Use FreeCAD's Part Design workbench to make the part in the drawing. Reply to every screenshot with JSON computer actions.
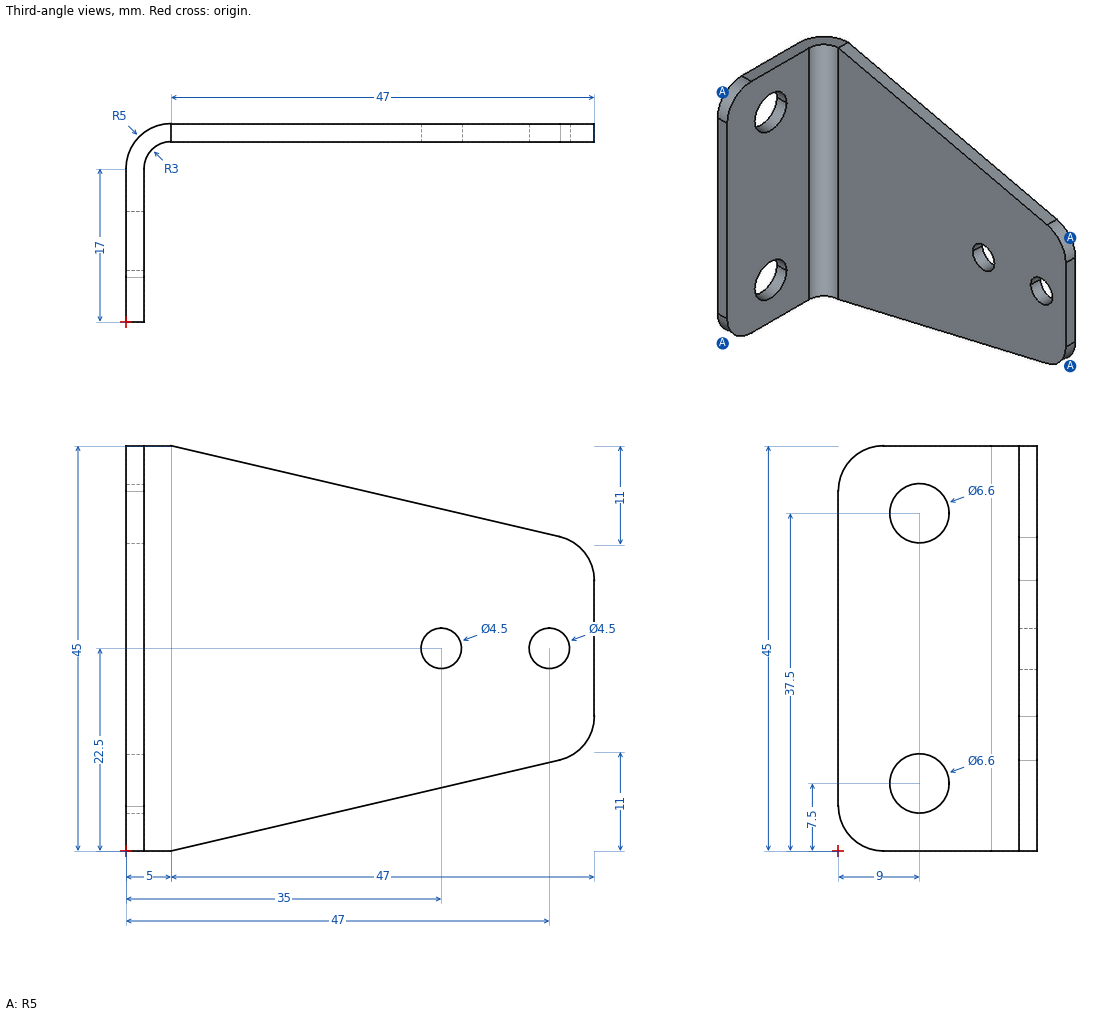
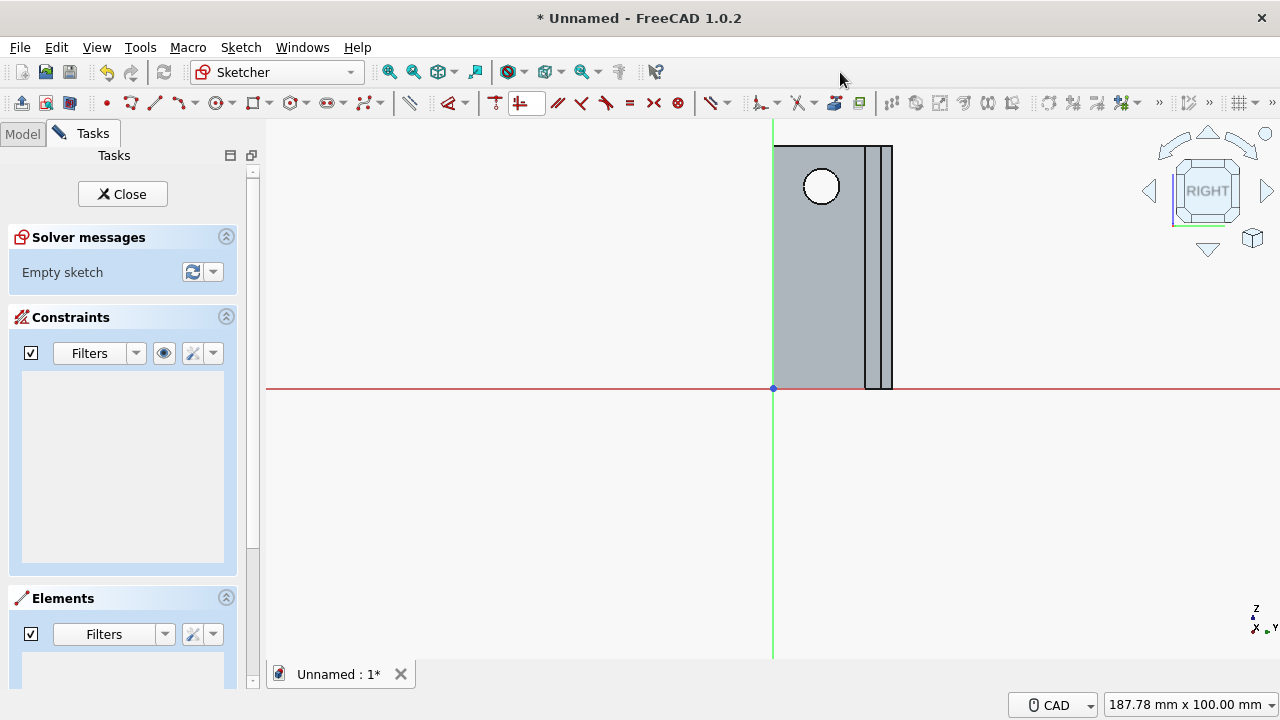
{"action": "scroll", "coordinate": [826, 354], "scroll_direction": "up", "scroll_amount": 9}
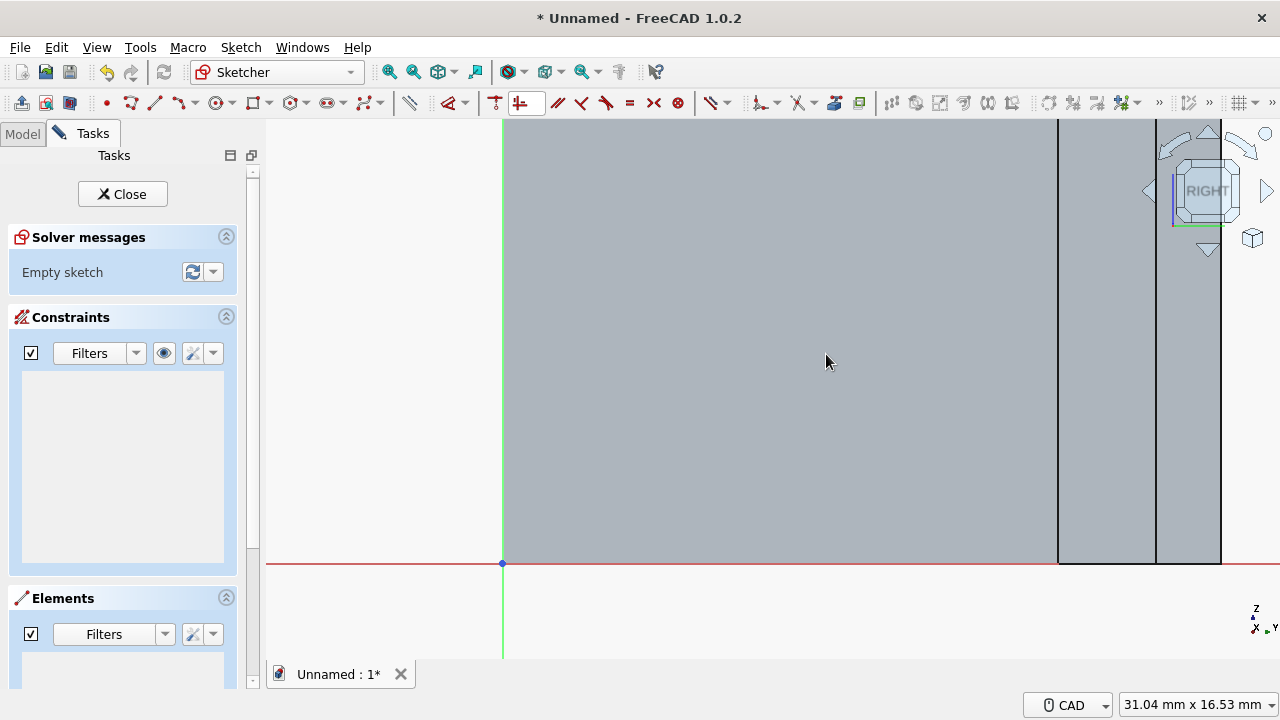
{"action": "key", "text": "g c"}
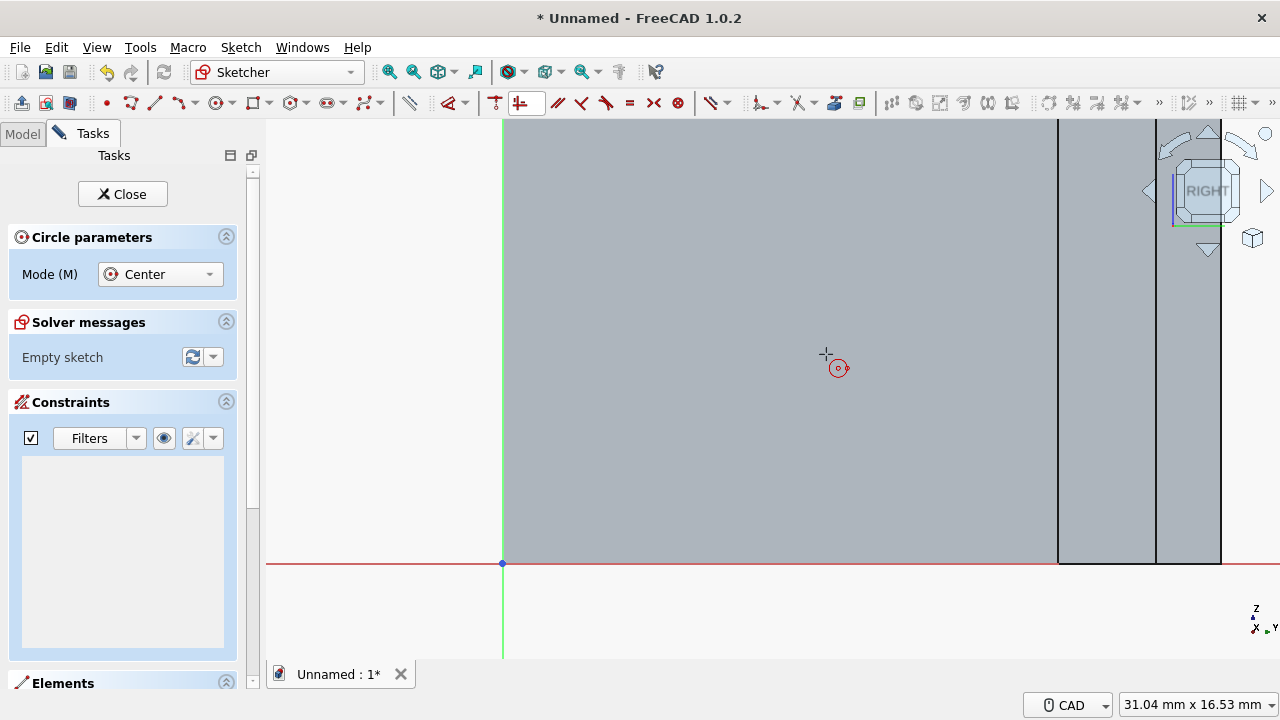
{"action": "left_click", "coordinate": [797, 319]}
{"action": "mouse_move", "coordinate": [873, 242]}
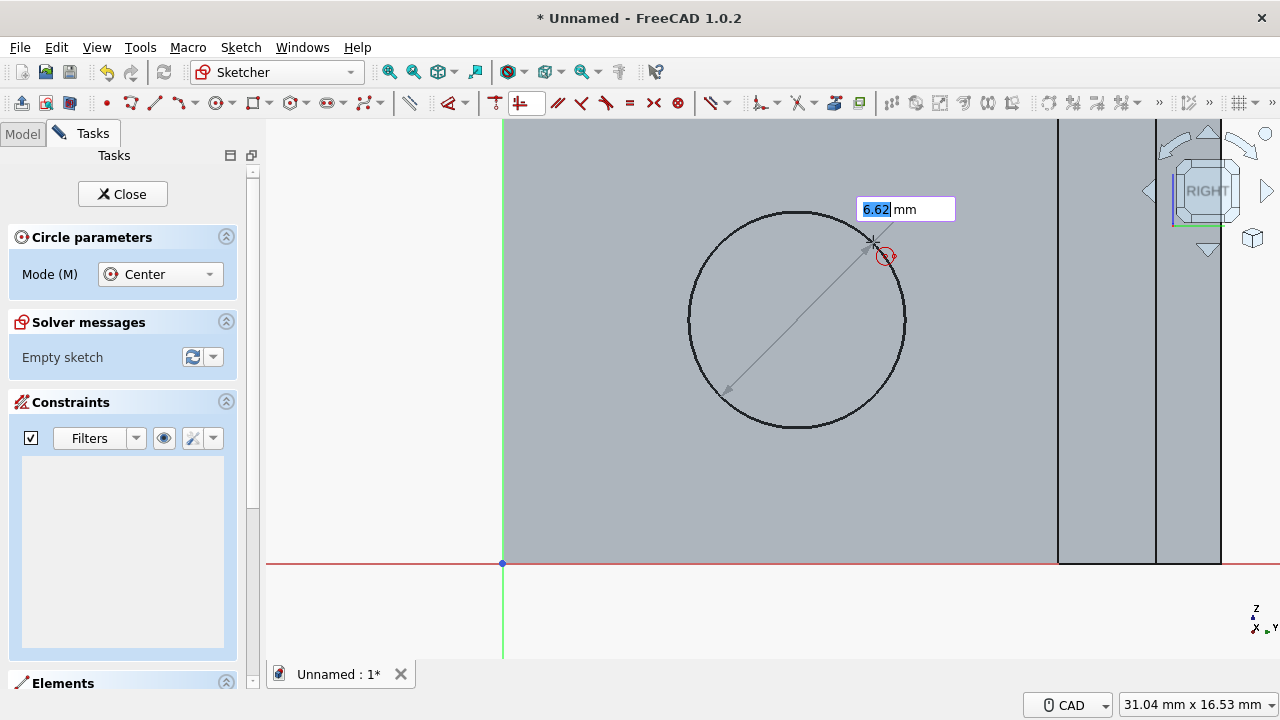
{"action": "type", "text": "6.6"}
{"action": "key", "text": "Return"}
{"action": "key", "text": "Escape"}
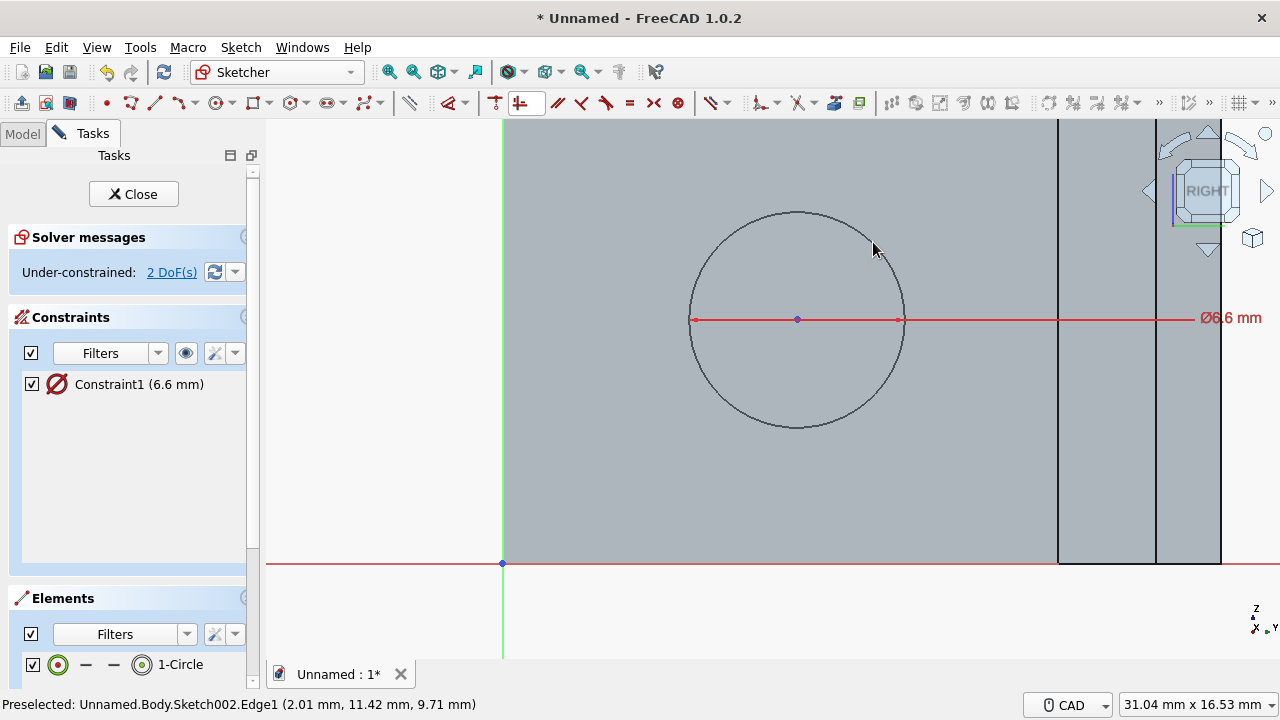
{"action": "key", "text": "d"}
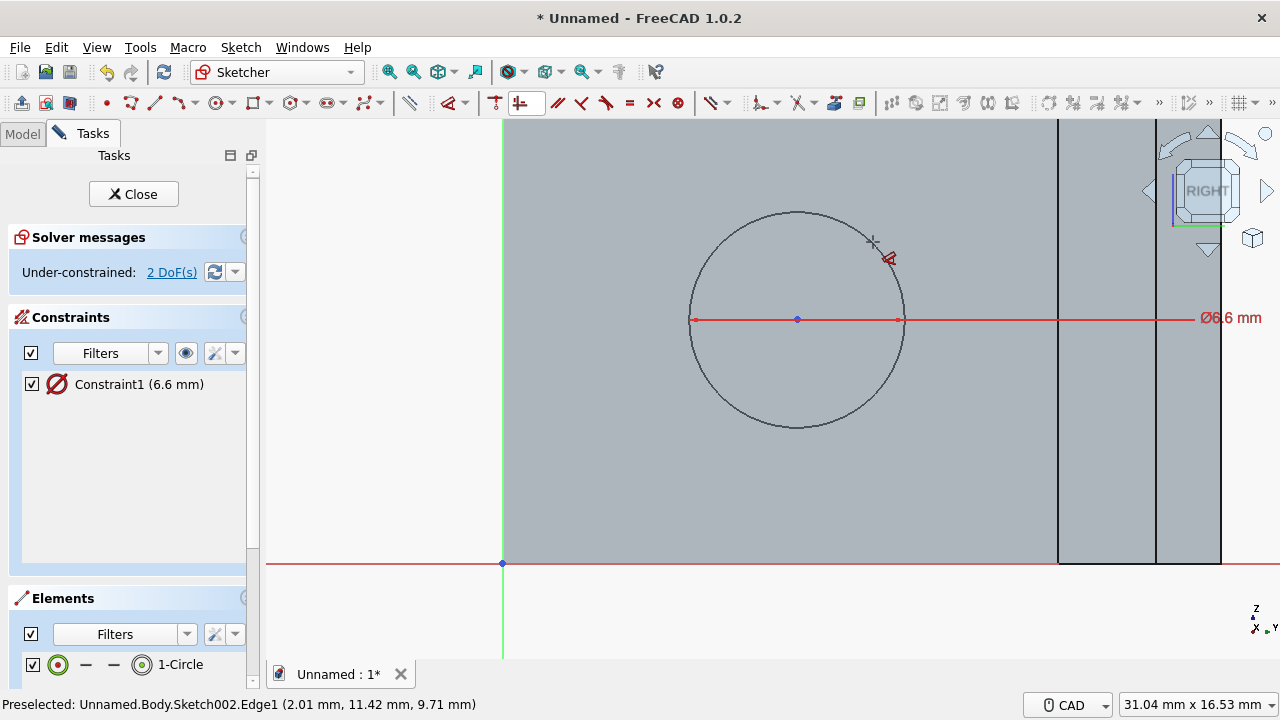
{"action": "left_click", "coordinate": [797, 320]}
{"action": "left_click", "coordinate": [650, 598]}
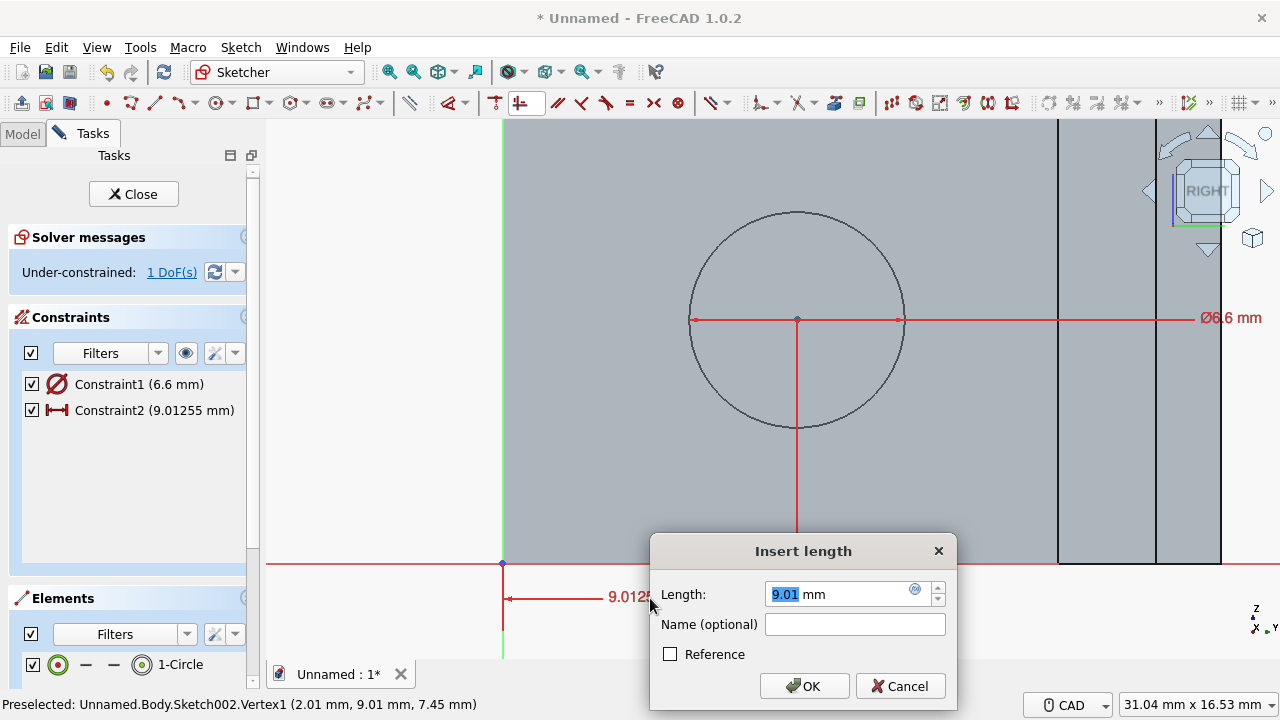
{"action": "type", "text": "9"}
{"action": "key", "text": "Return"}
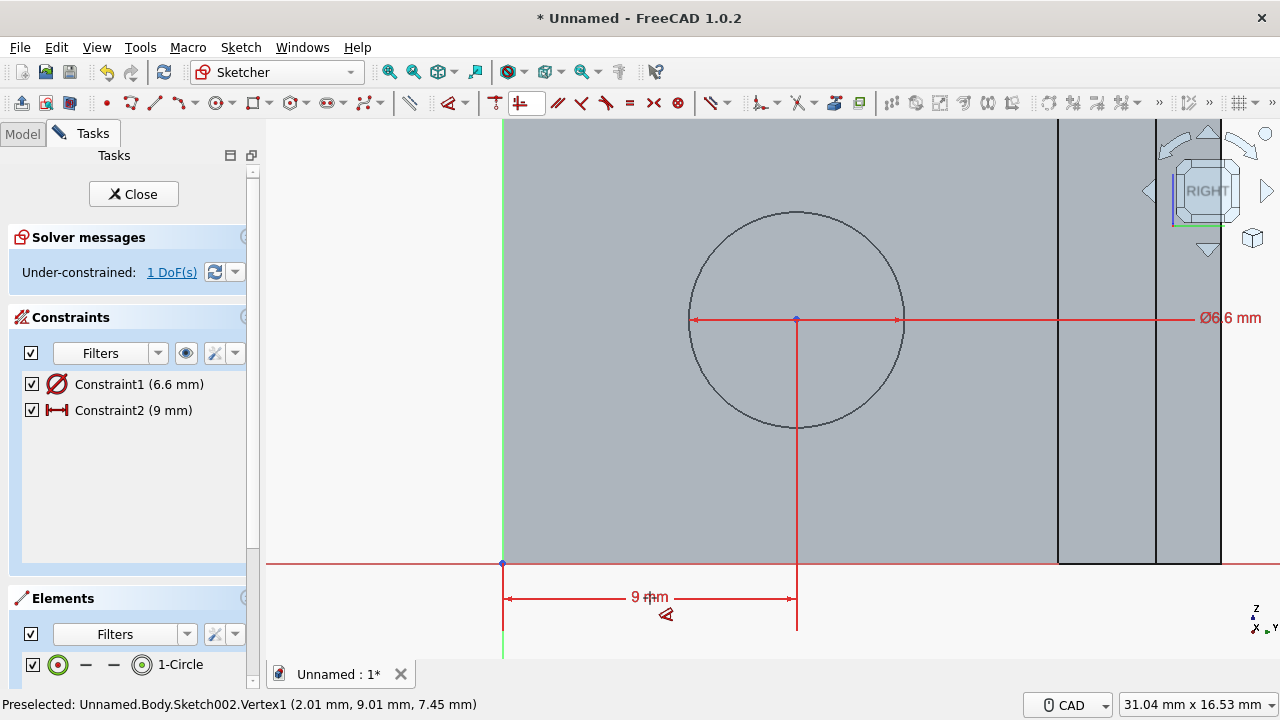
{"action": "left_click", "coordinate": [797, 320]}
{"action": "left_click", "coordinate": [469, 442]}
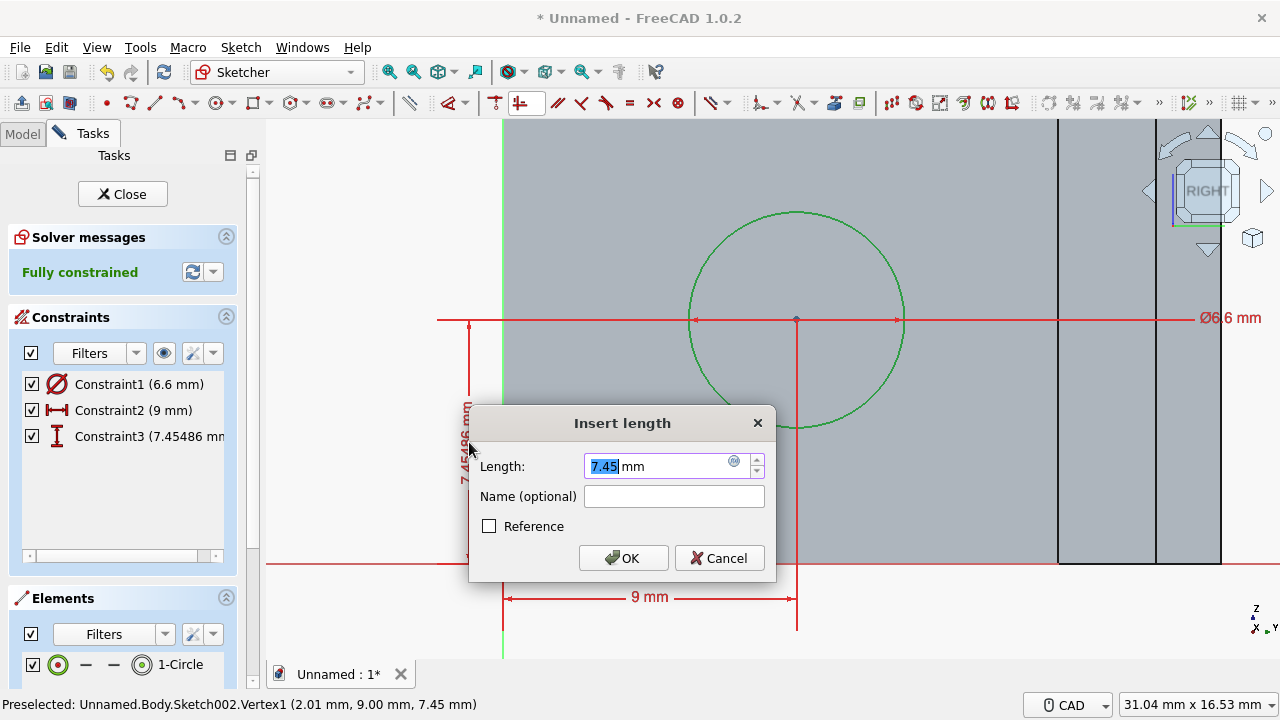
{"action": "type", "text": "7.5"}
{"action": "key", "text": "Return"}
{"action": "key", "text": "Escape"}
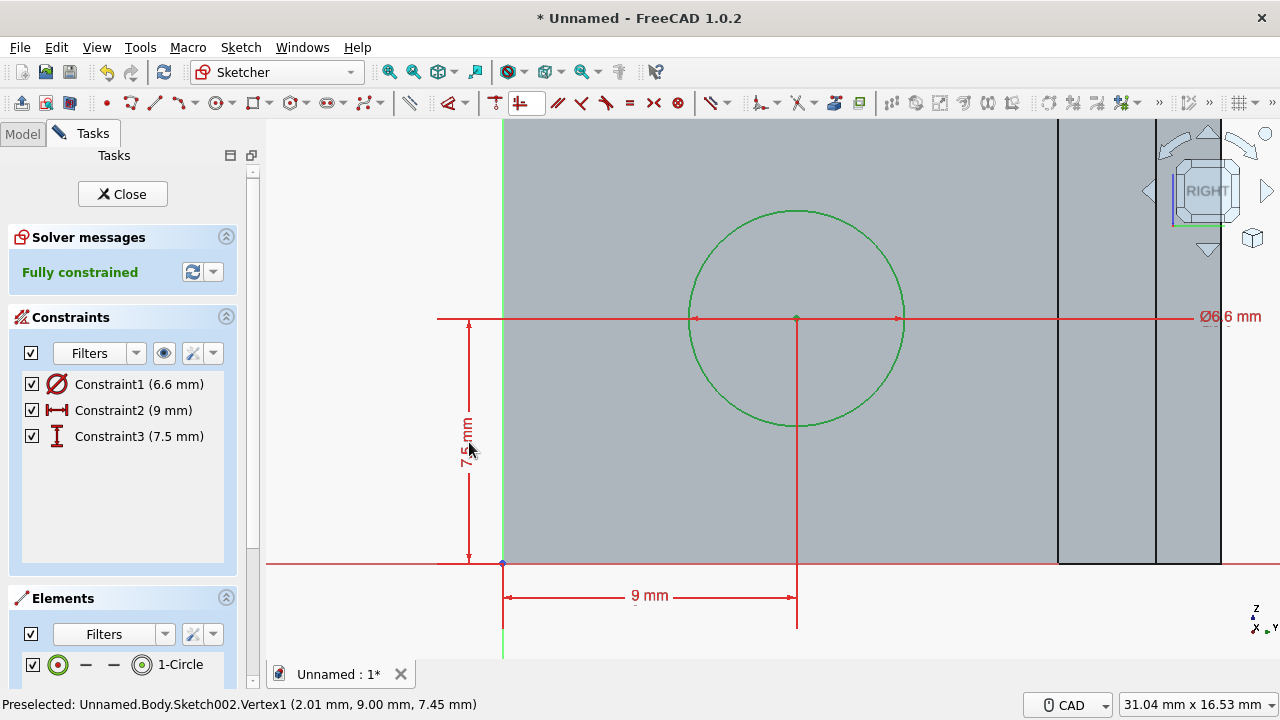
{"action": "left_click", "coordinate": [123, 194]}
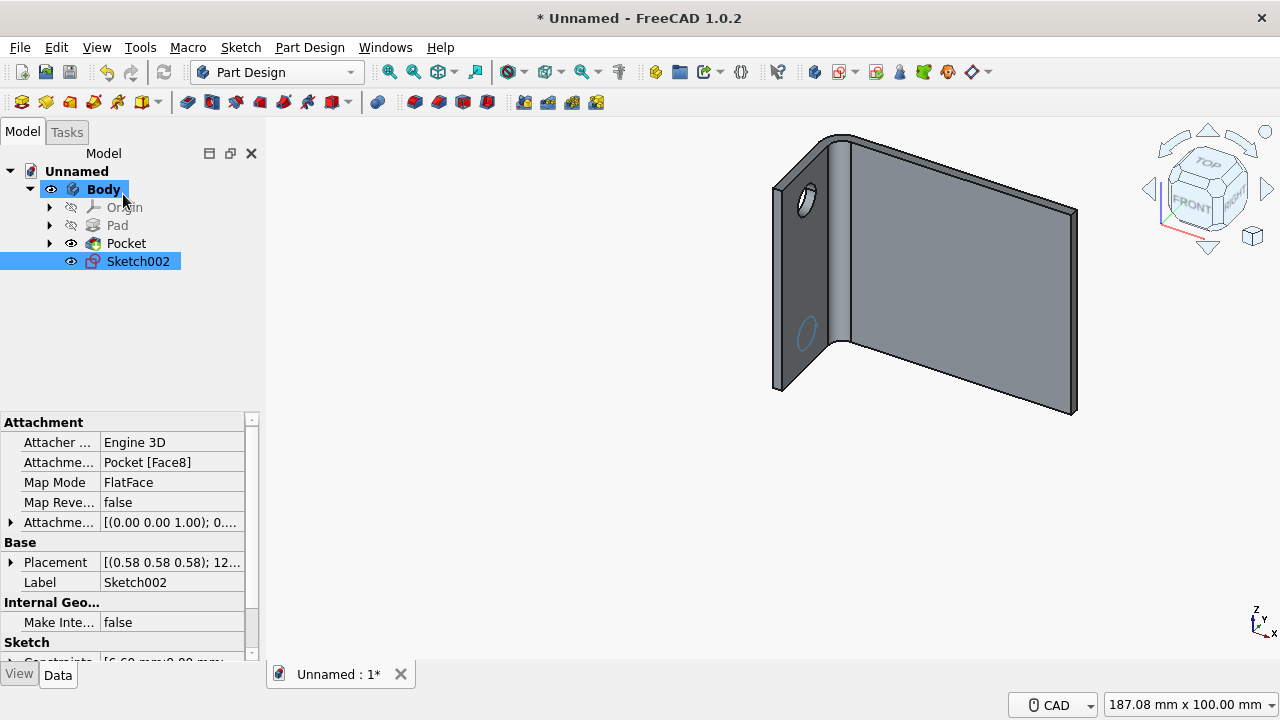
{"action": "left_click", "coordinate": [188, 102]}